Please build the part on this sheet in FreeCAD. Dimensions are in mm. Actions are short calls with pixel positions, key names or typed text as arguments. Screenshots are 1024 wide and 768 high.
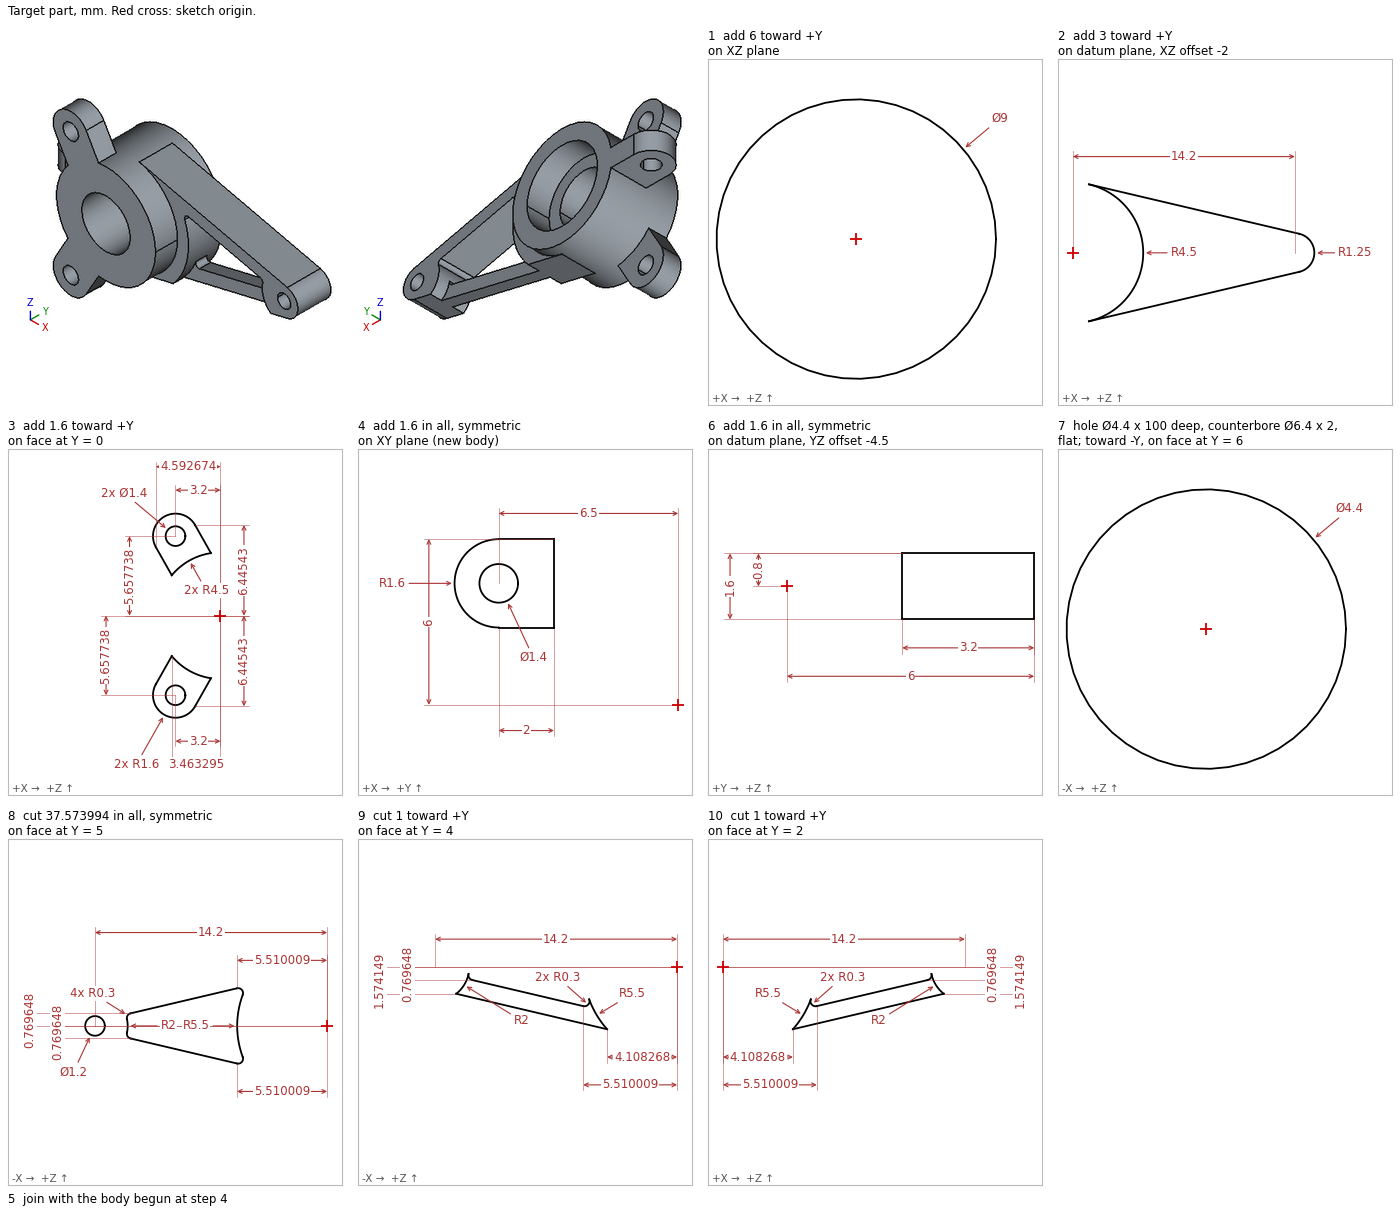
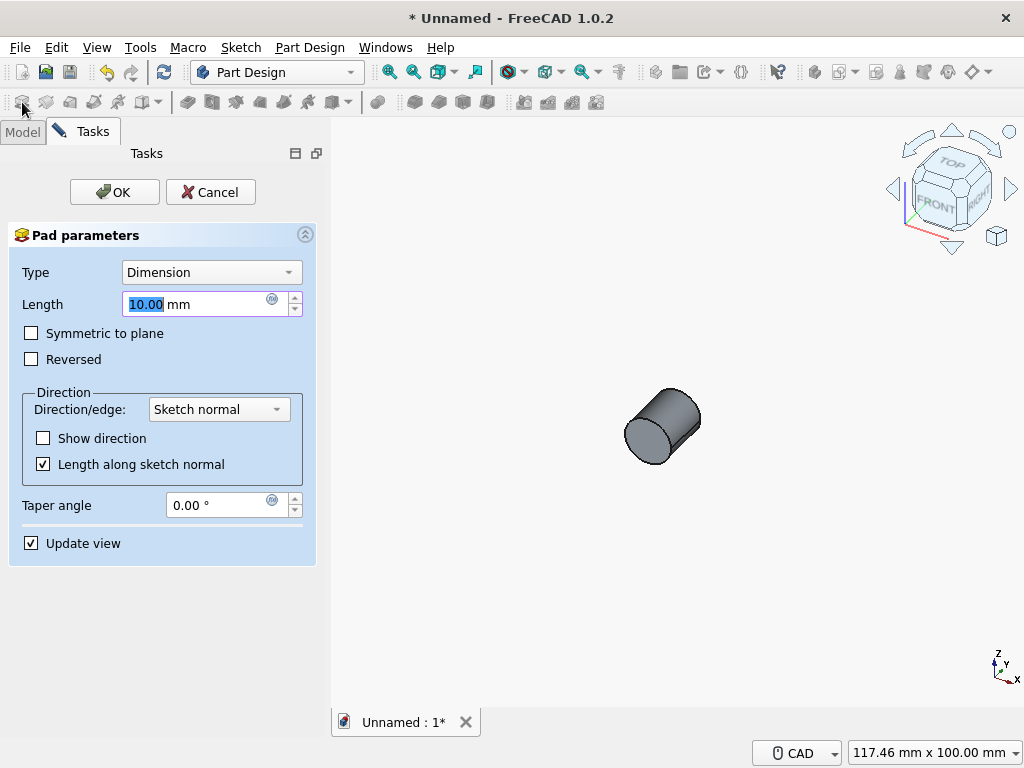
text(6)
key(Tab)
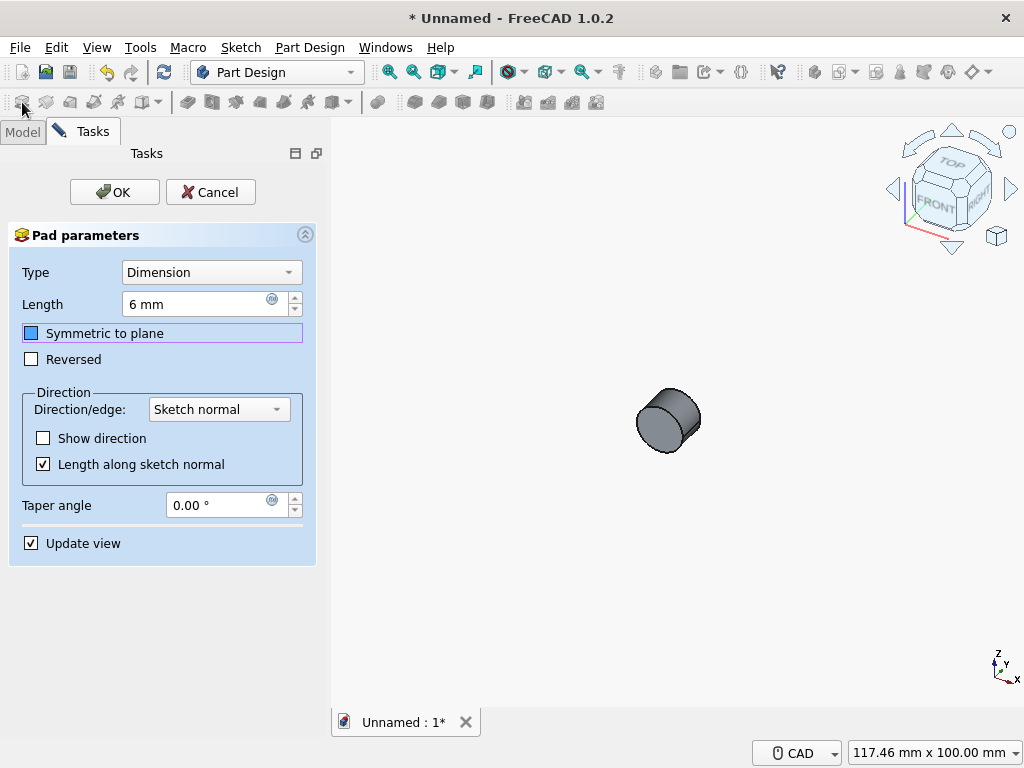
click(30, 359)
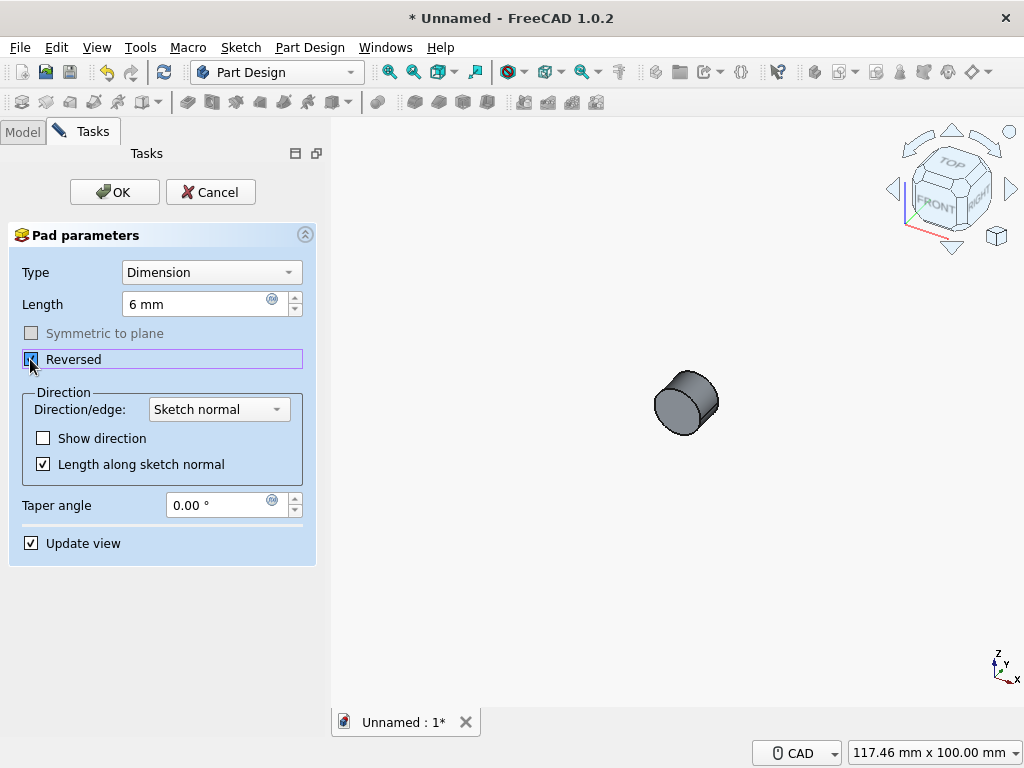
click(115, 192)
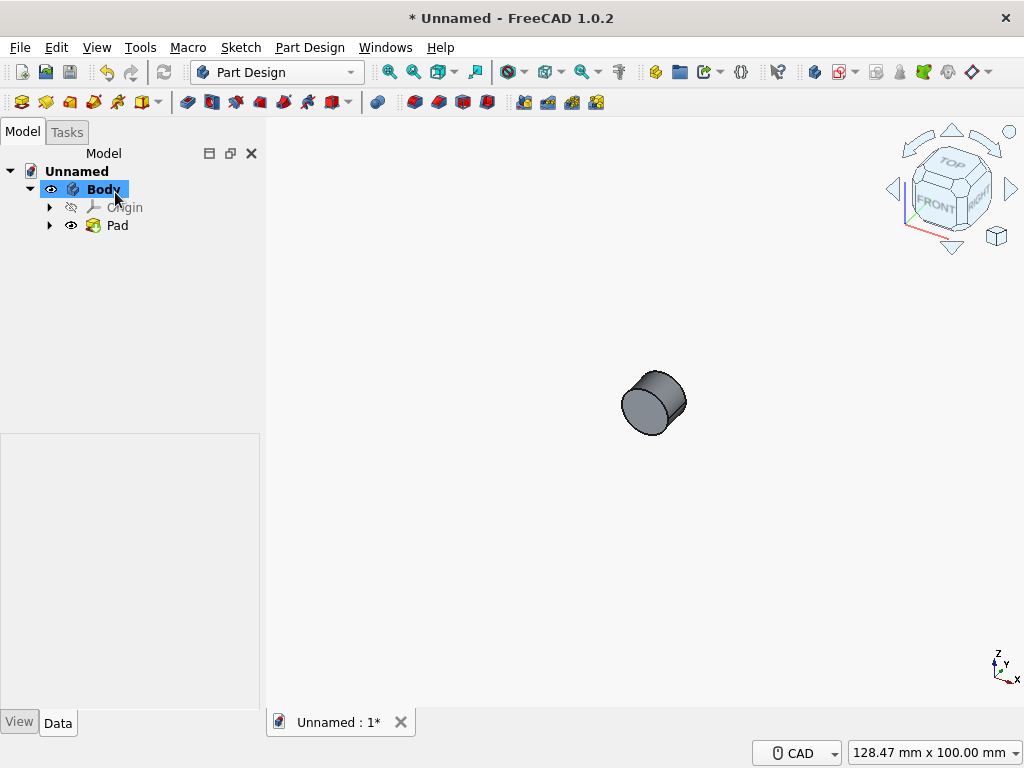
key(v)
key(f)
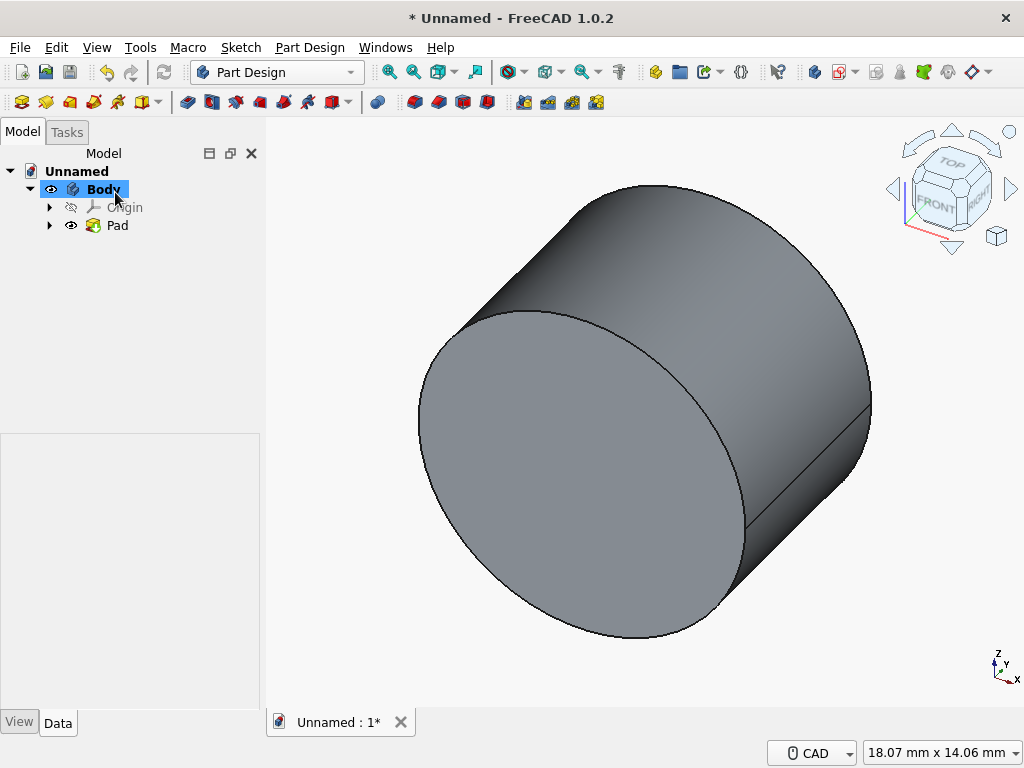
click(50, 207)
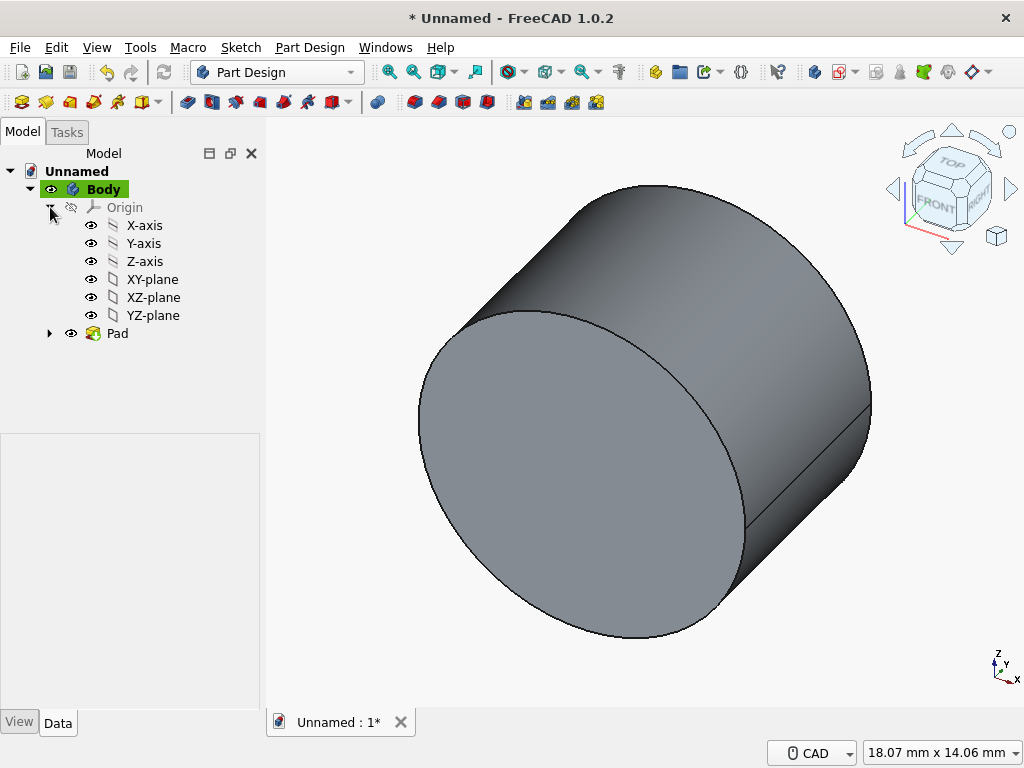
click(136, 297)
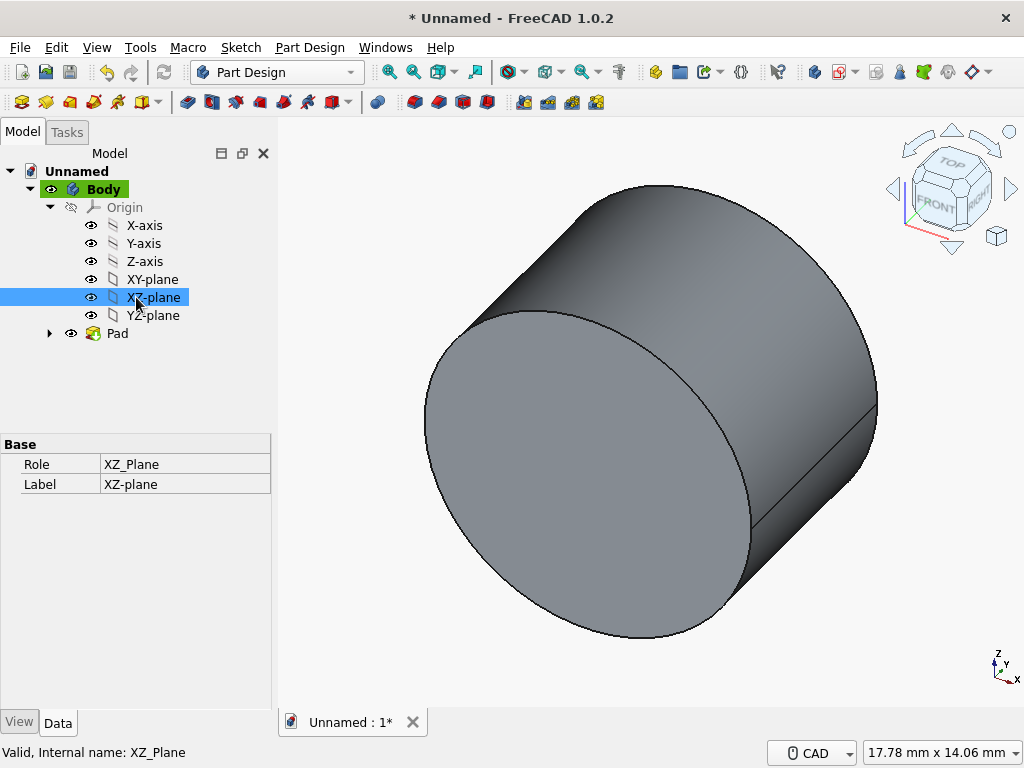
click(972, 72)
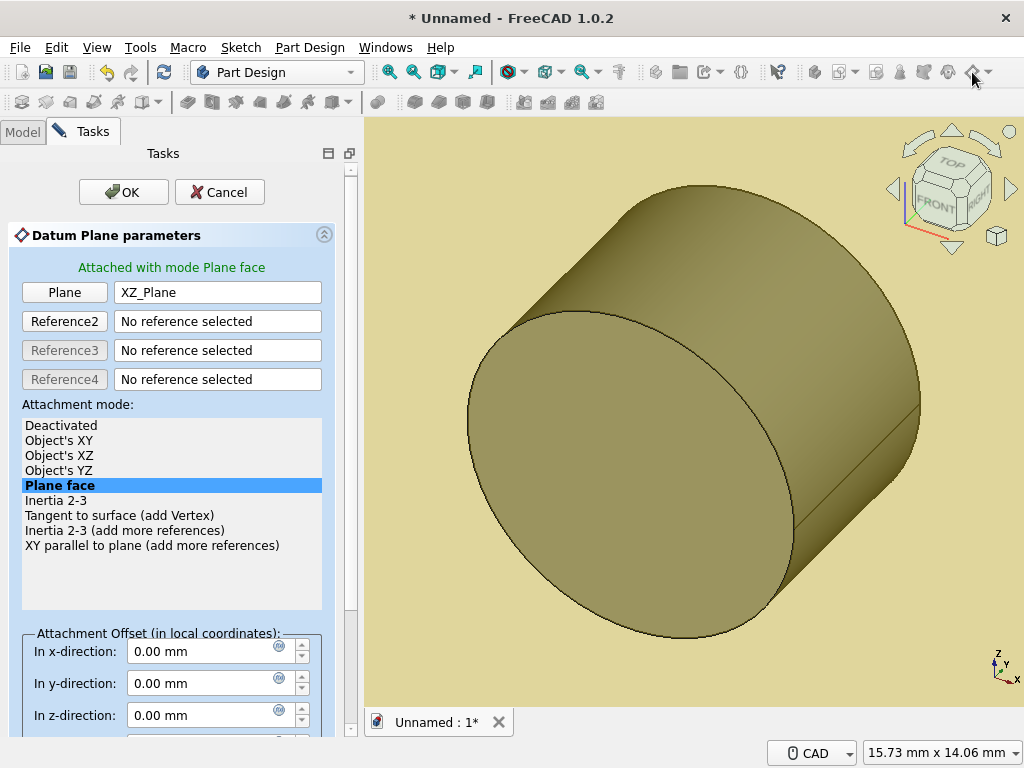
triple_click(210, 715)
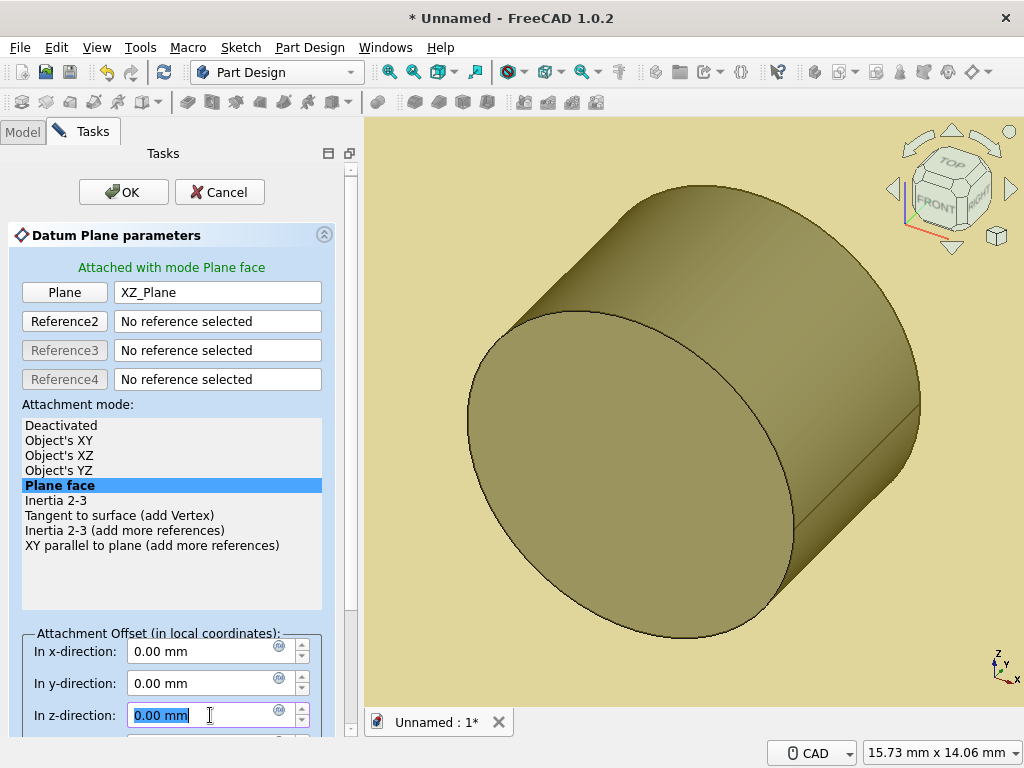
text(-2)
key(Tab)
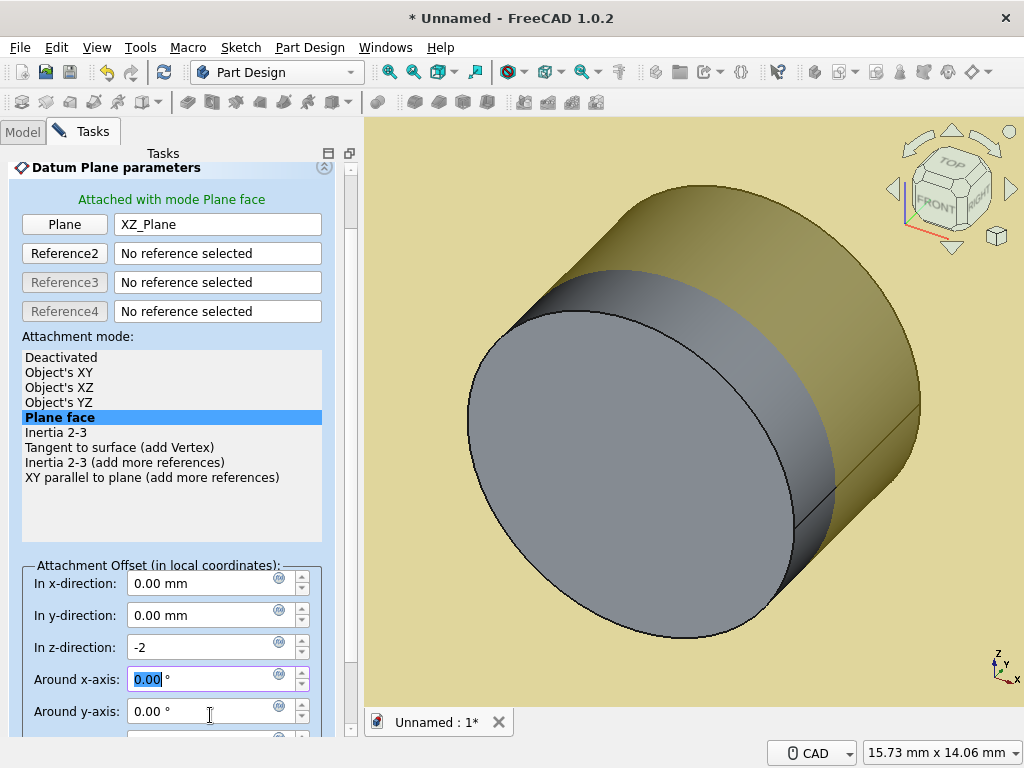
scroll(351, 450, up, 2)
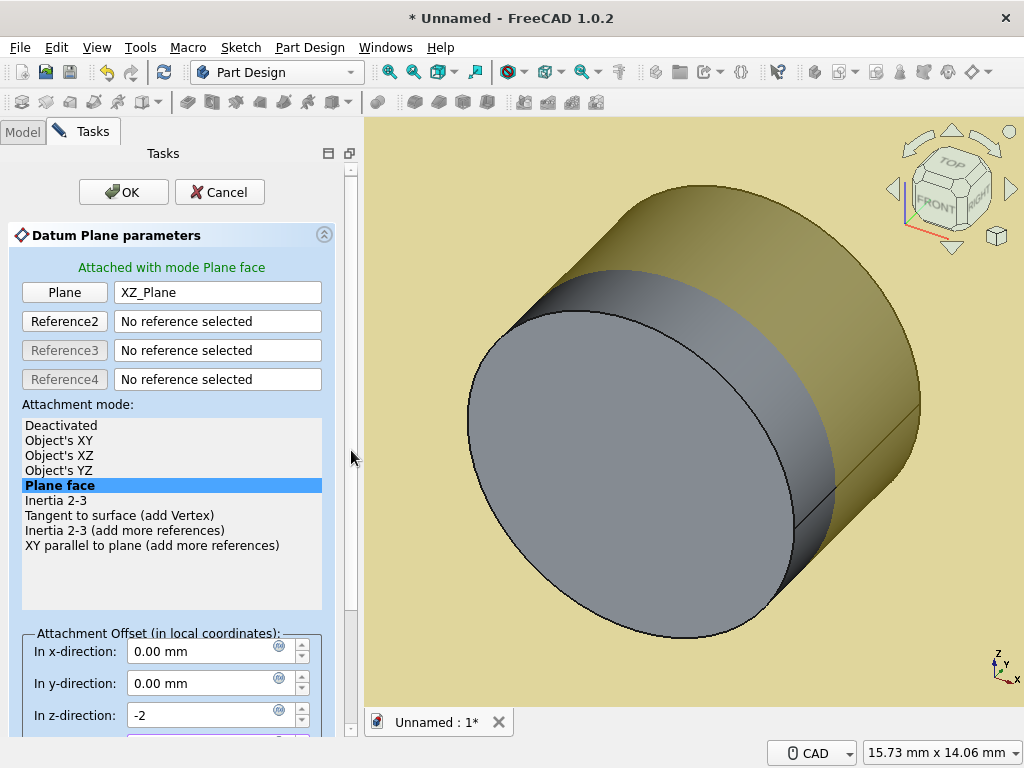
click(124, 192)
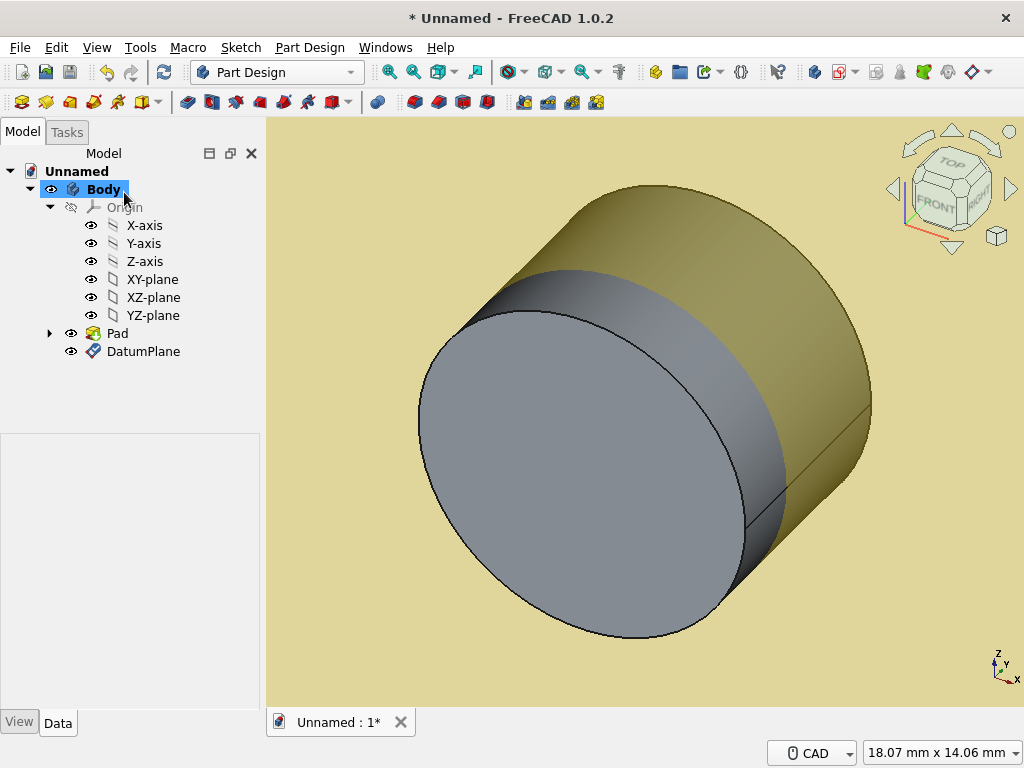
click(116, 351)